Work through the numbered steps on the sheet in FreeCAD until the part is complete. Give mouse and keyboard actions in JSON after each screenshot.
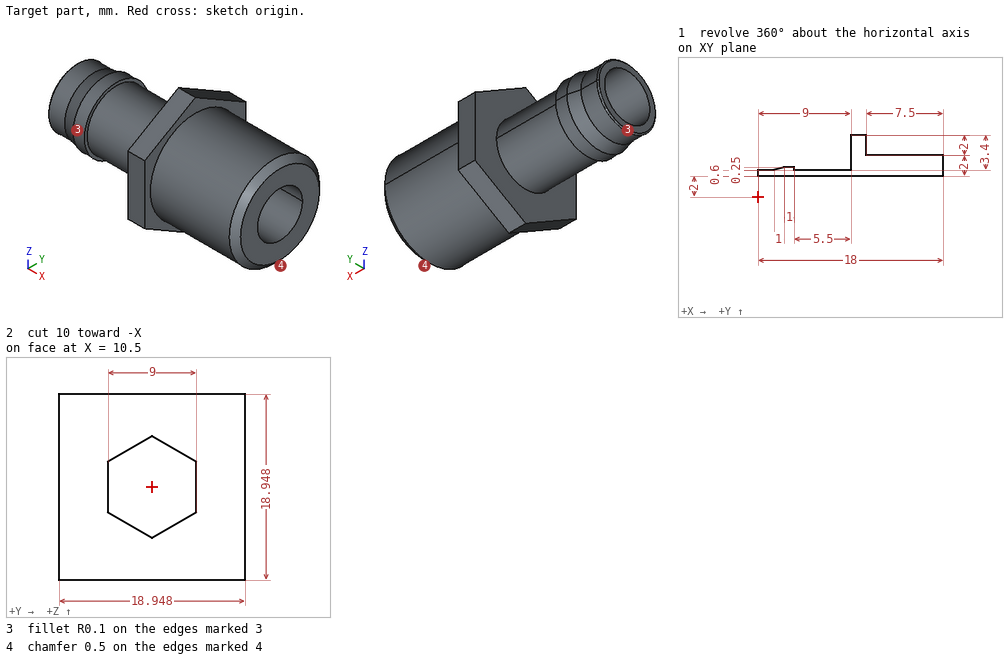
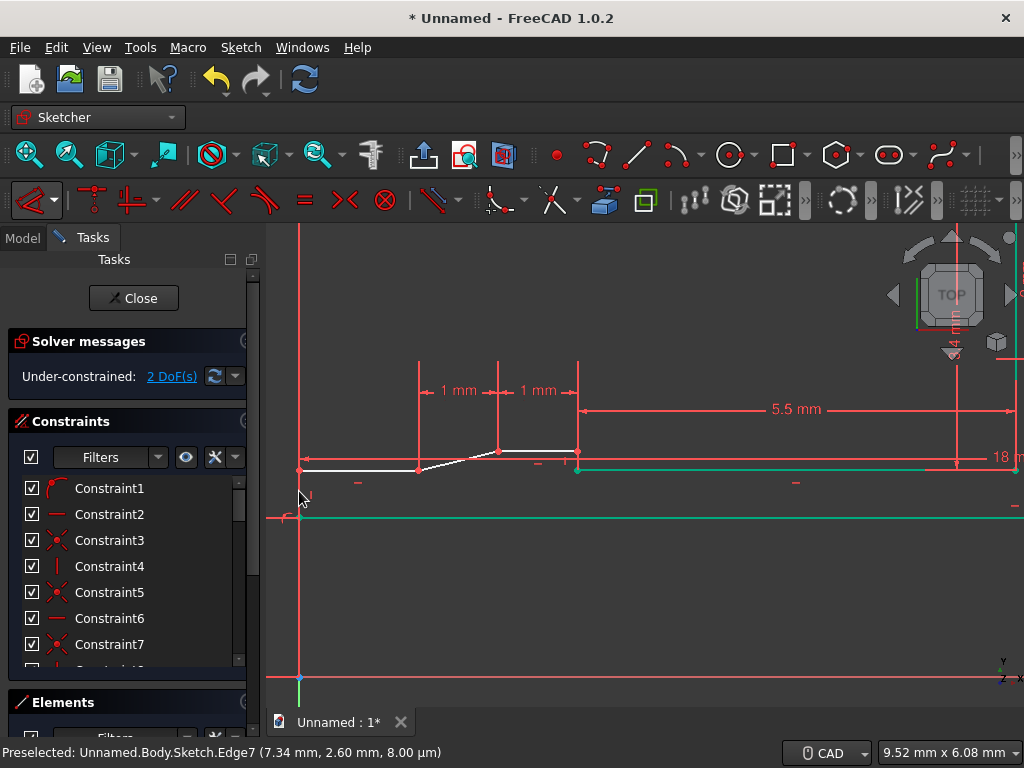
{"action": "left_click", "coordinate": [299, 490]}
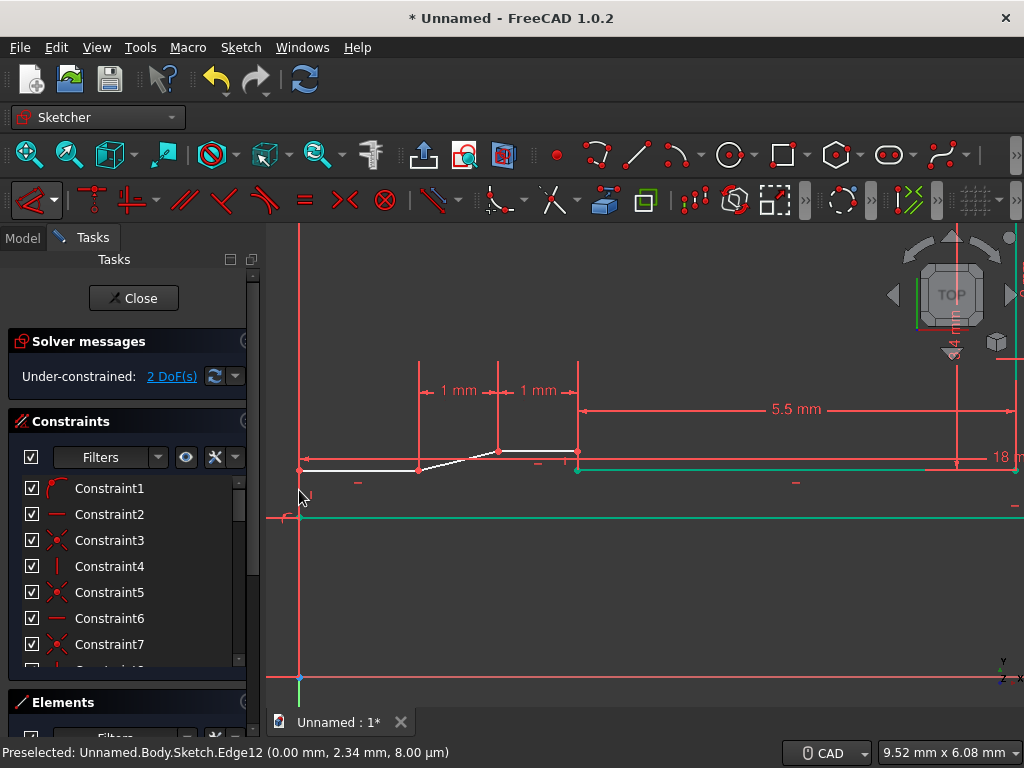
{"action": "key", "text": "i"}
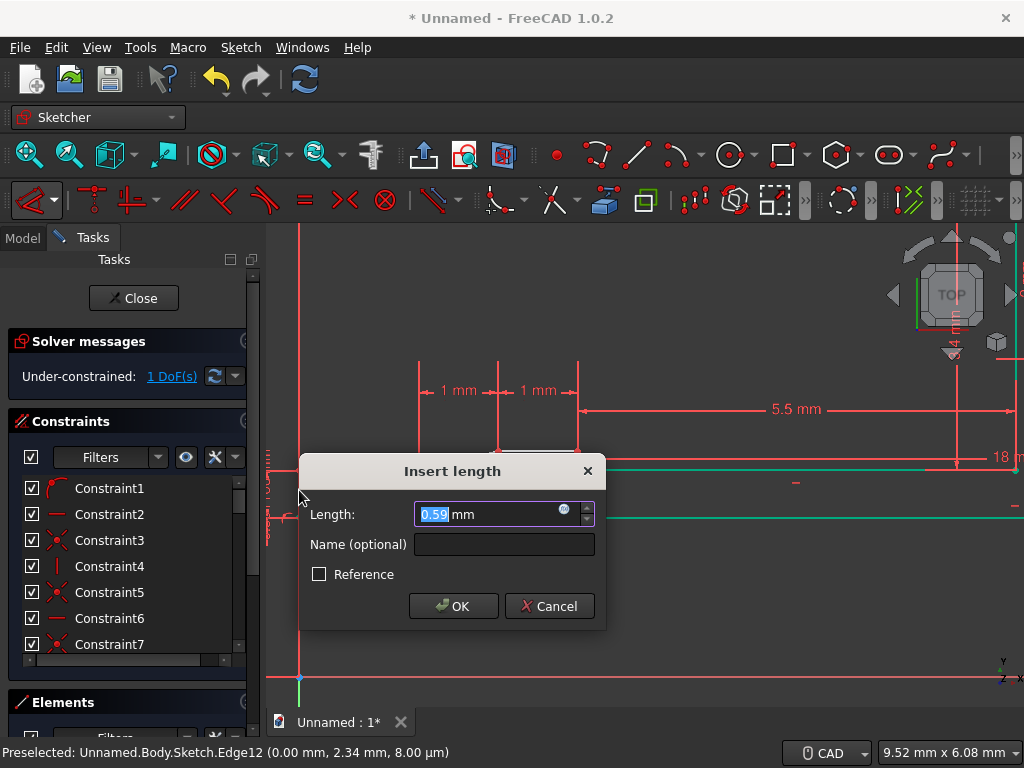
{"action": "type", "text": "0.6"}
{"action": "key", "text": "Return"}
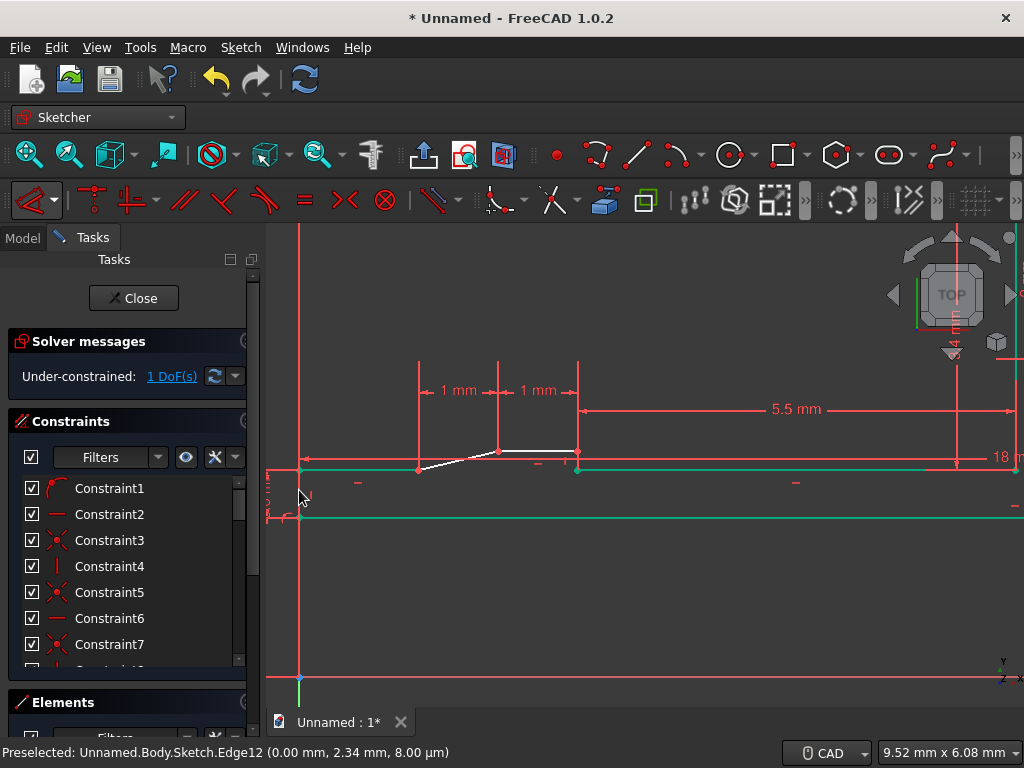
{"action": "scroll", "coordinate": [578, 461], "scroll_direction": "up", "scroll_amount": 4}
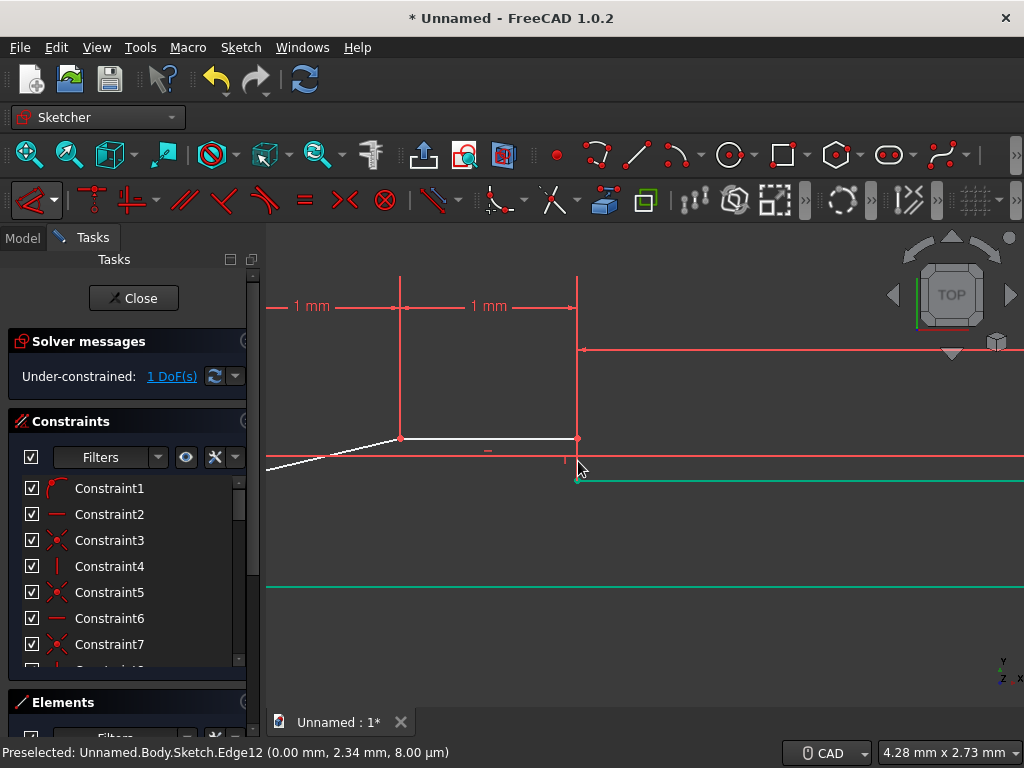
{"action": "left_click", "coordinate": [577, 460]}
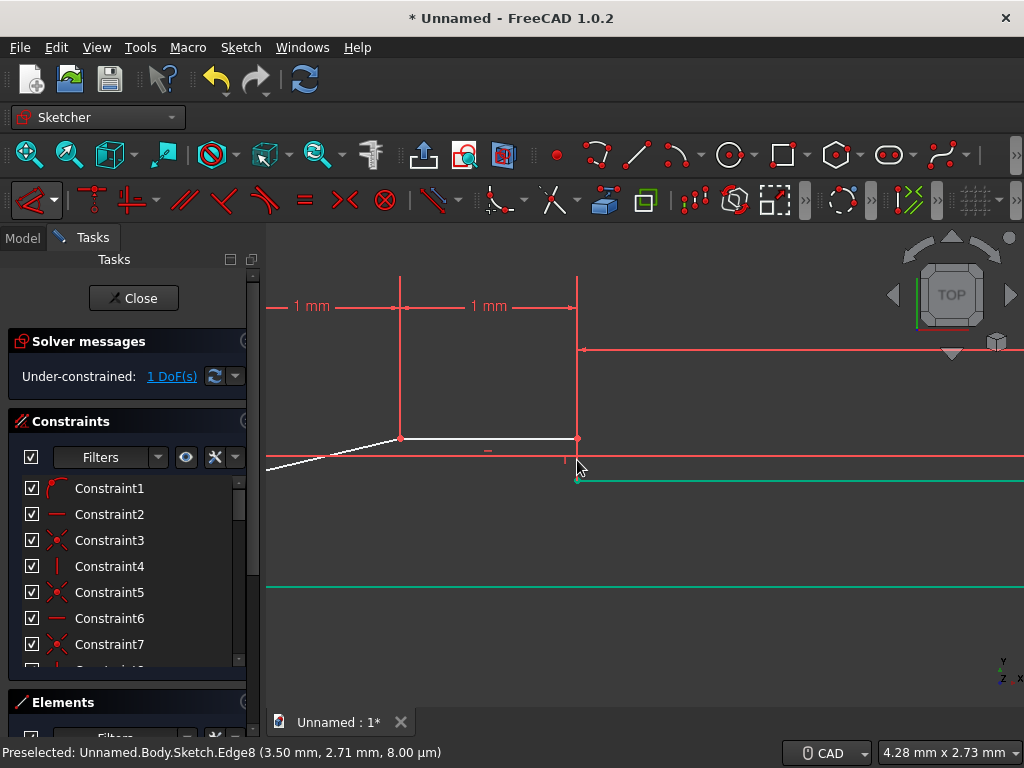
{"action": "key", "text": "i"}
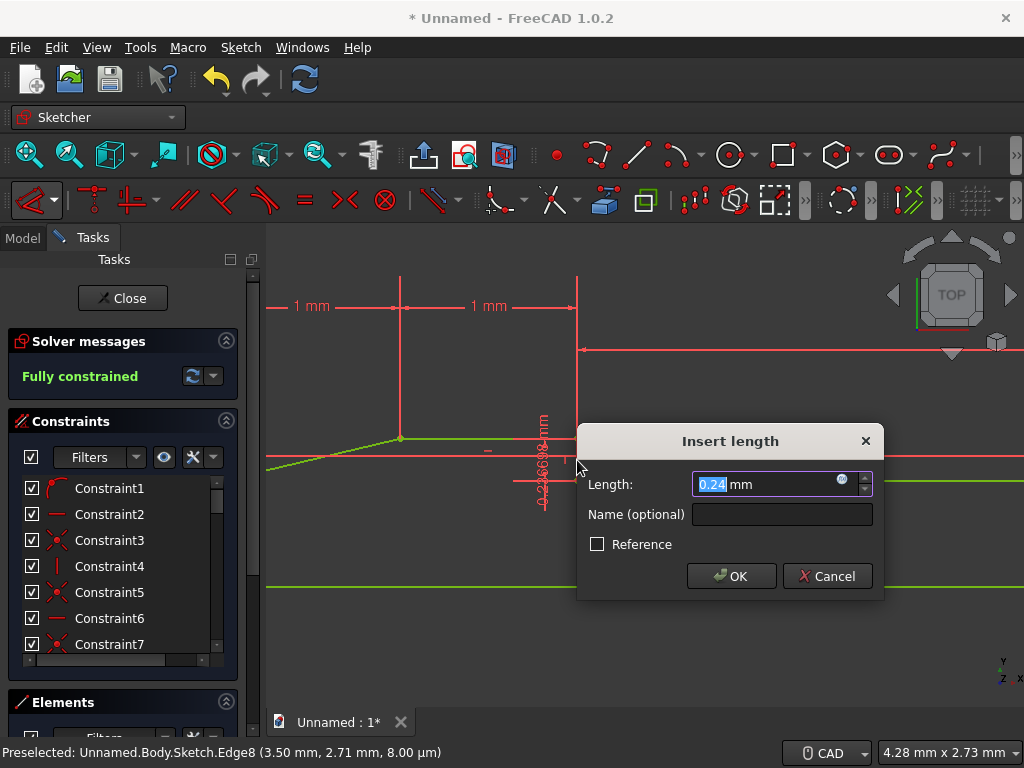
{"action": "type", "text": "0.25"}
{"action": "key", "text": "Return"}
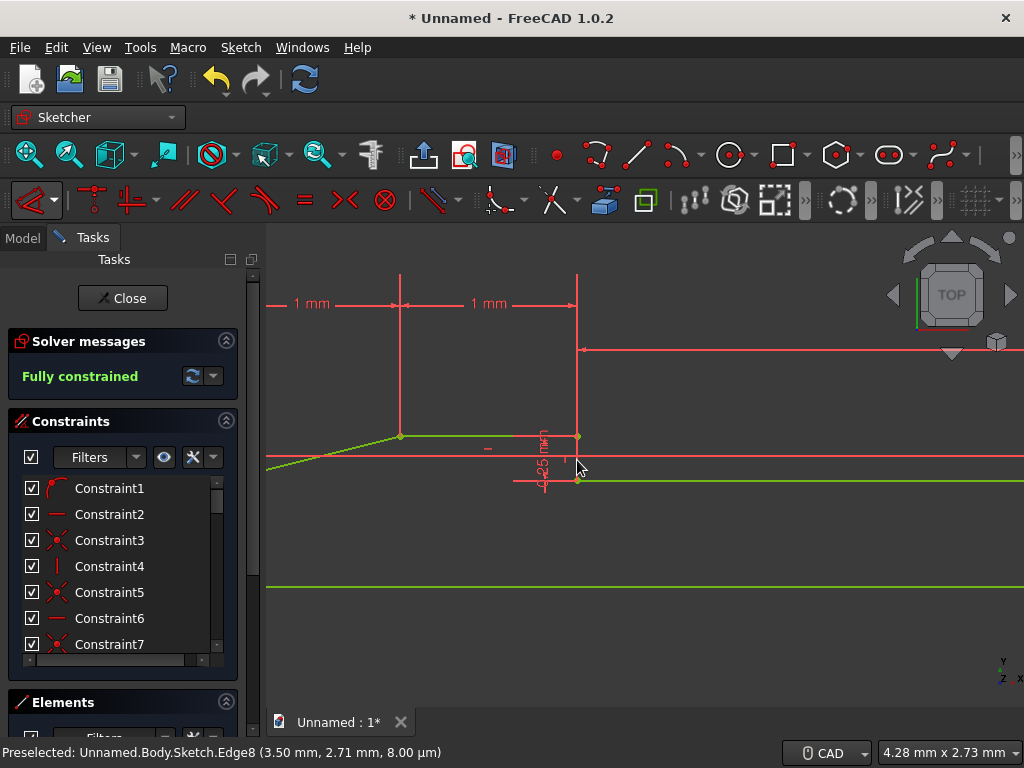
{"action": "left_click", "coordinate": [123, 298]}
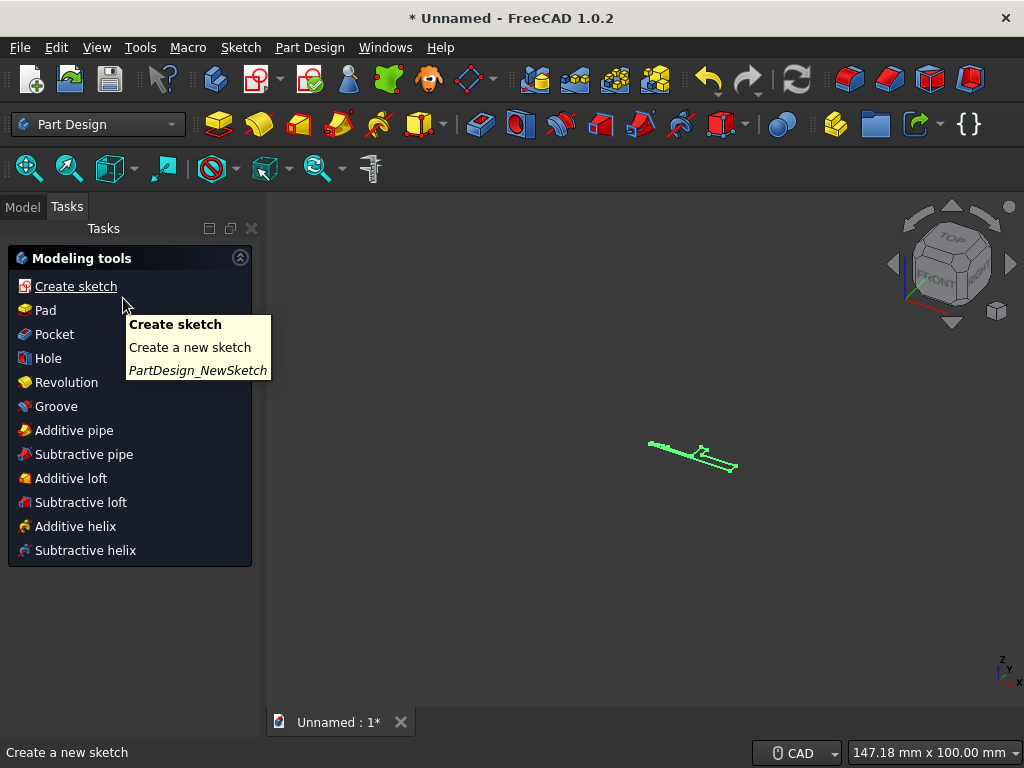
{"action": "left_click", "coordinate": [260, 124]}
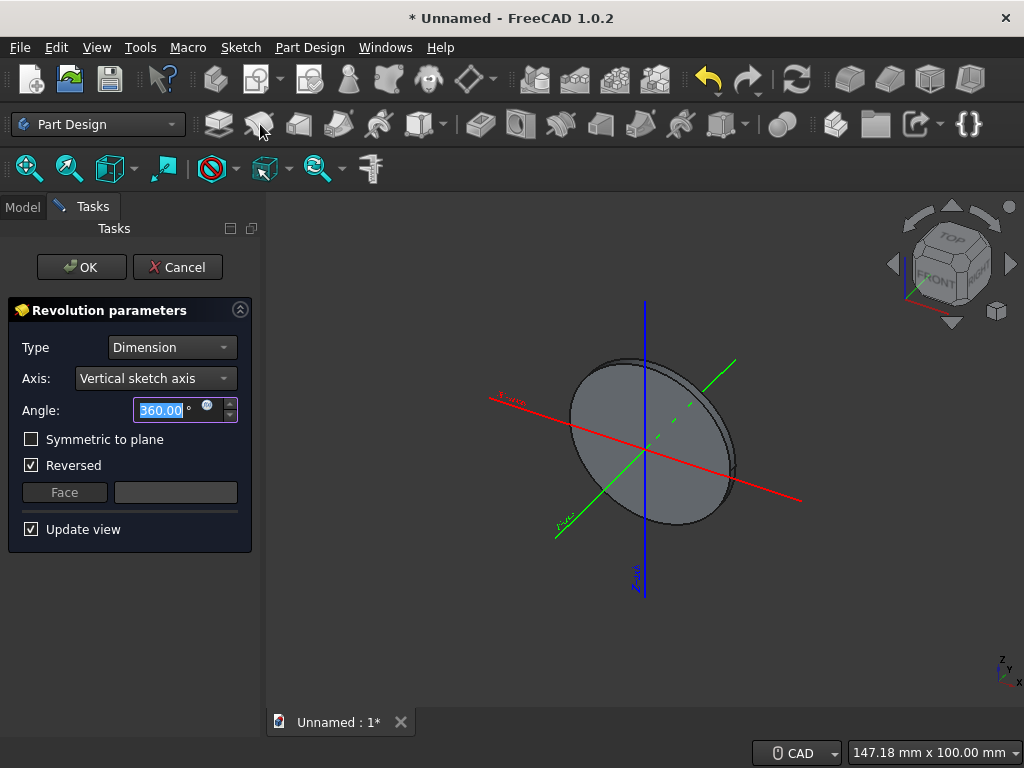
{"action": "left_click", "coordinate": [156, 378]}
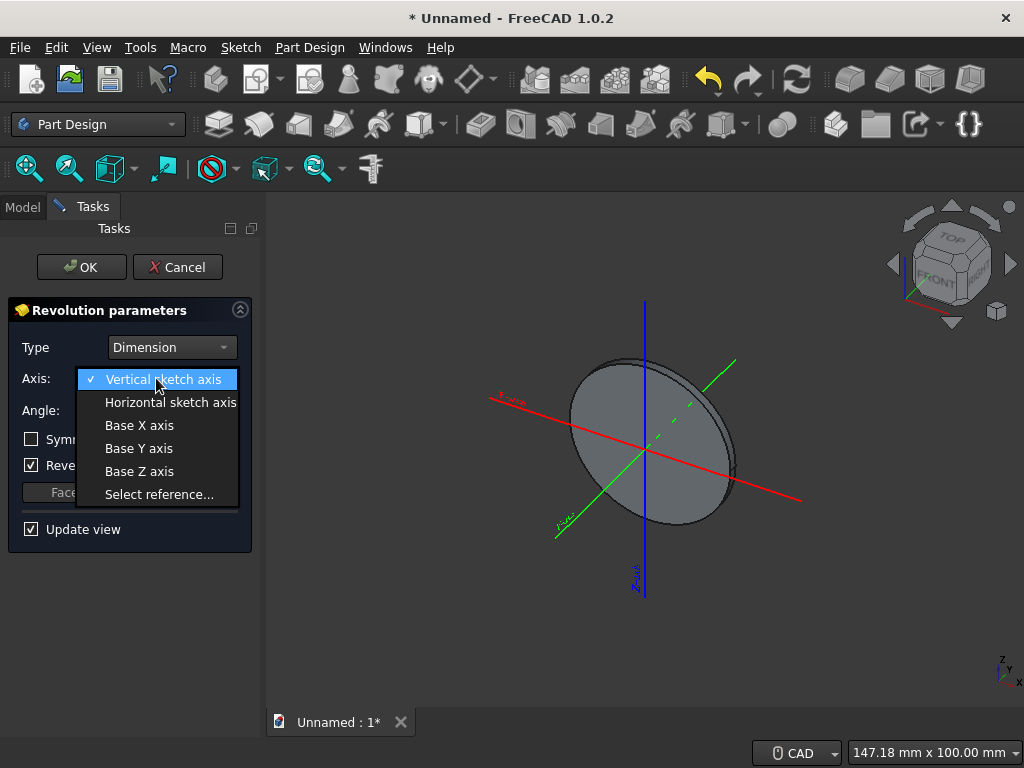
{"action": "left_click", "coordinate": [156, 402]}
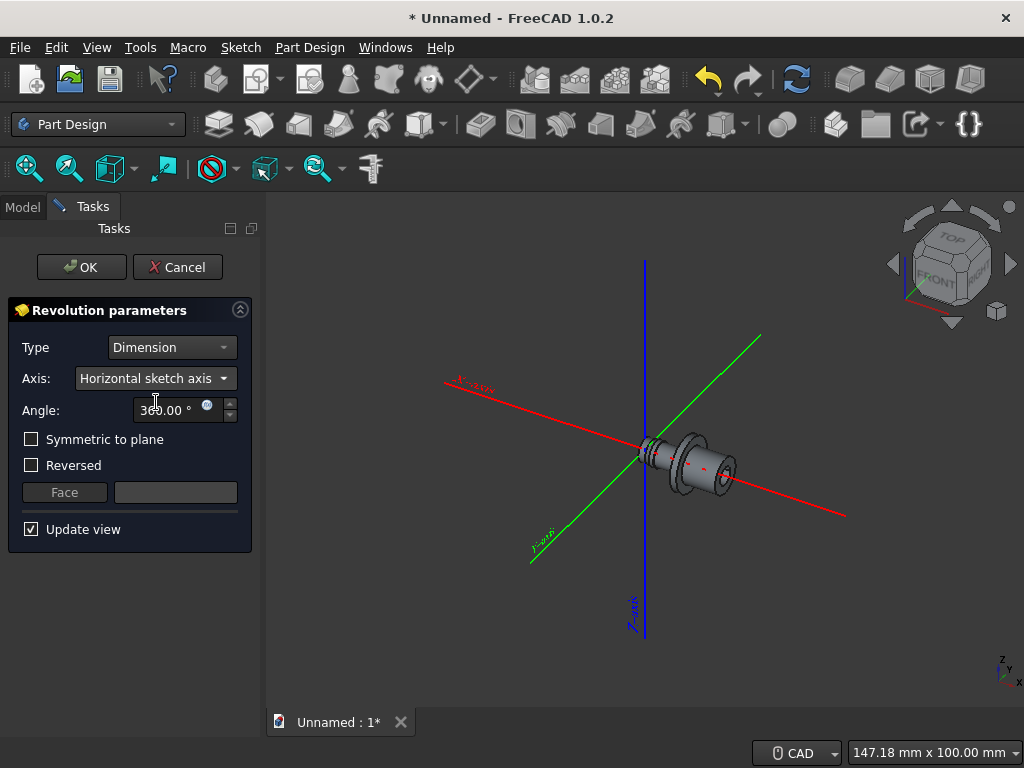
{"action": "left_click", "coordinate": [82, 267]}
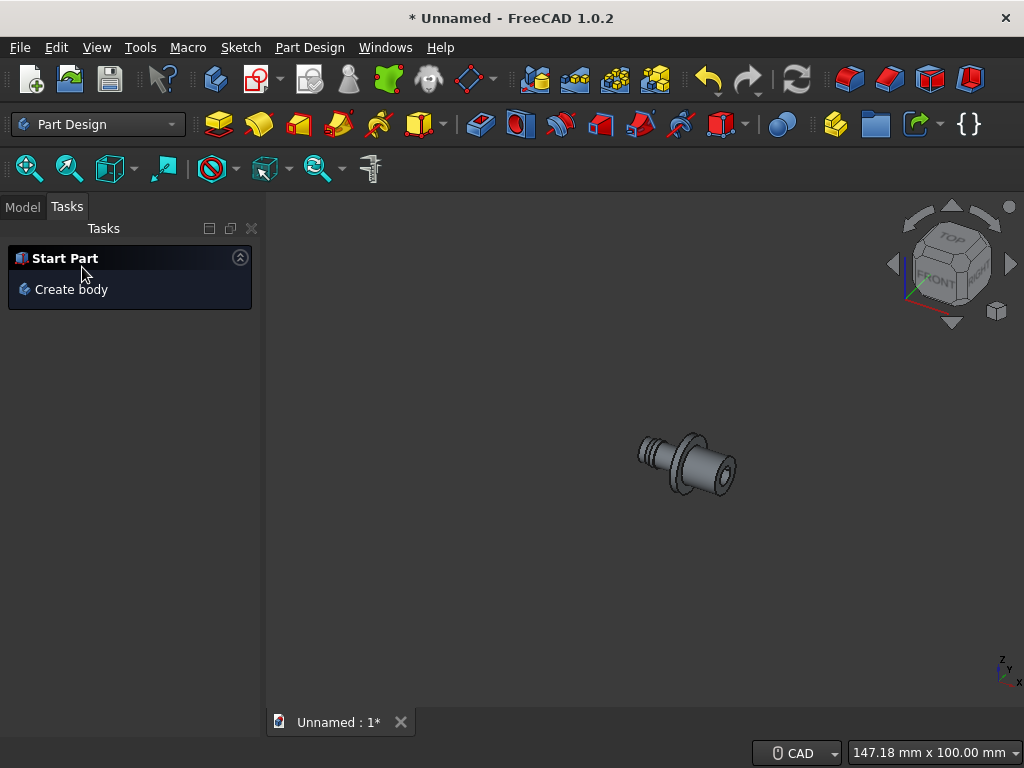
{"action": "left_click", "coordinate": [30, 170]}